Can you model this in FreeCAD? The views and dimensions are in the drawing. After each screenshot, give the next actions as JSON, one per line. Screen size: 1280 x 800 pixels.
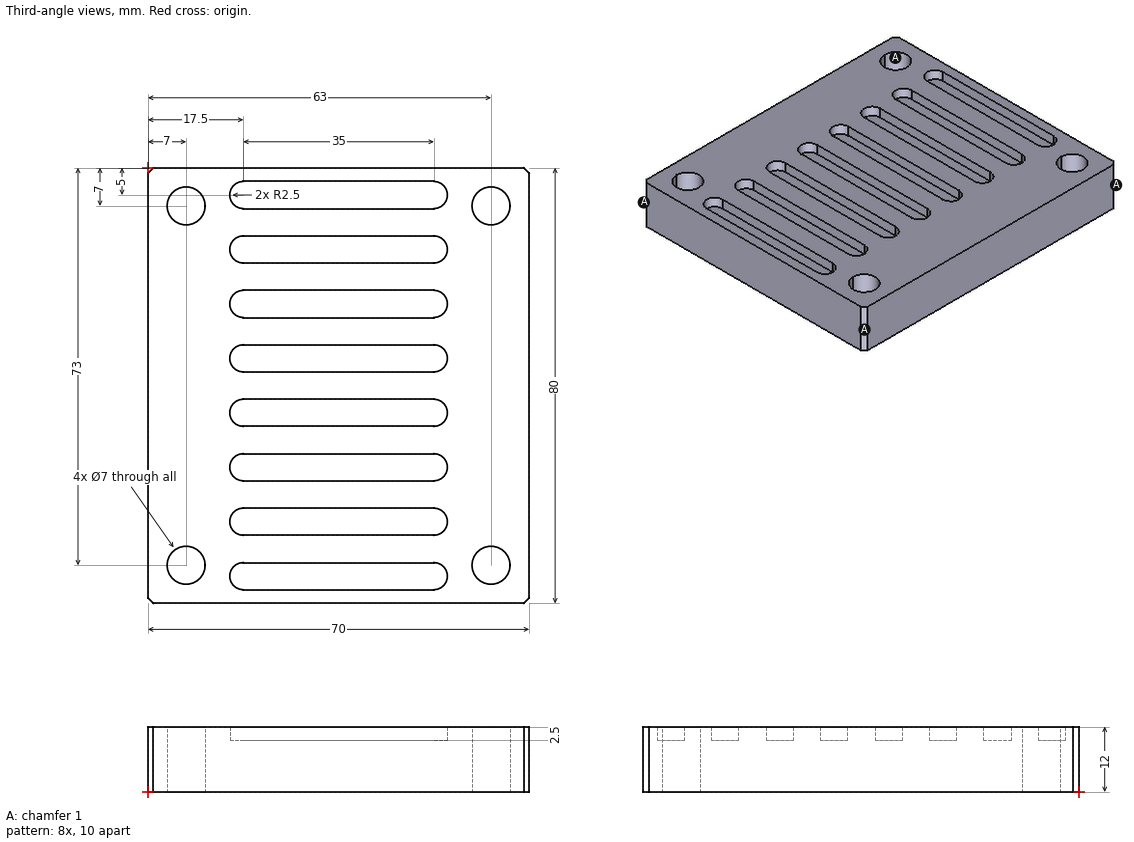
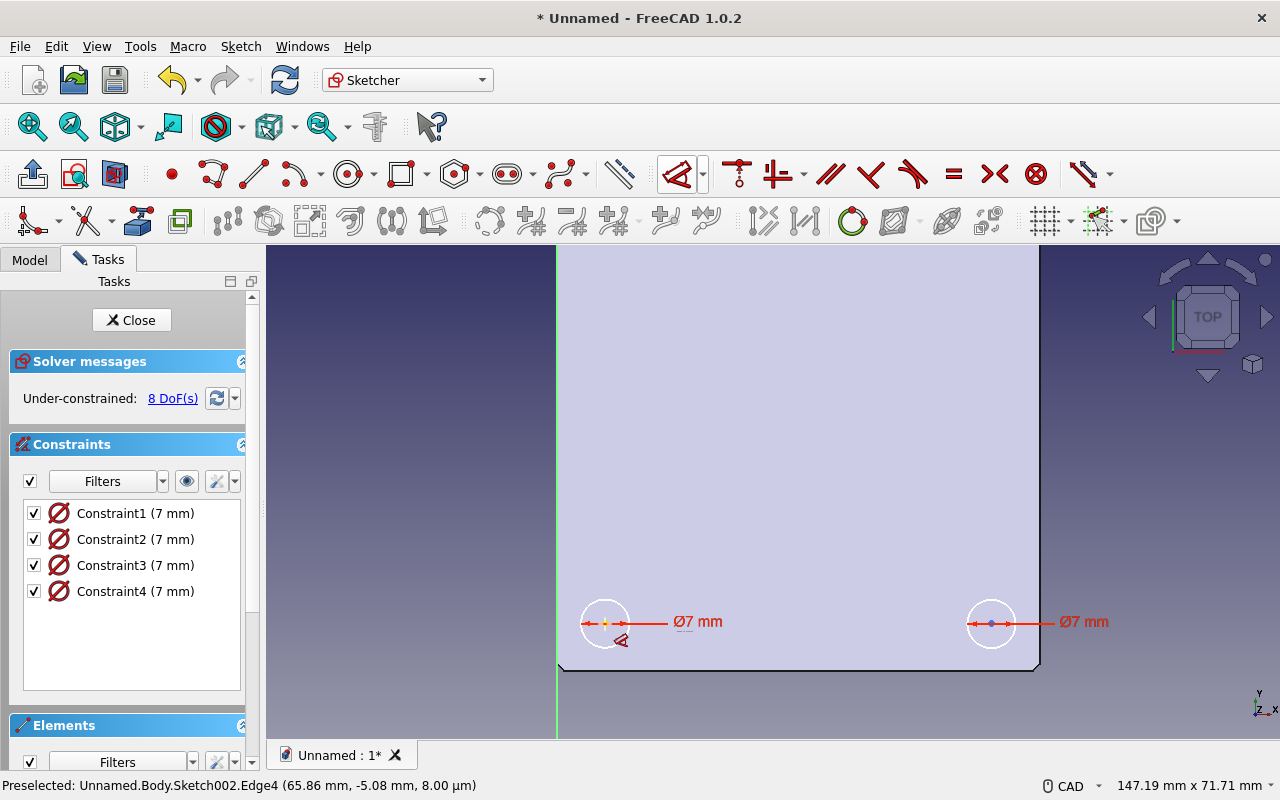
{"action": "left_click", "coordinate": [605, 624]}
{"action": "left_click", "coordinate": [581, 658]}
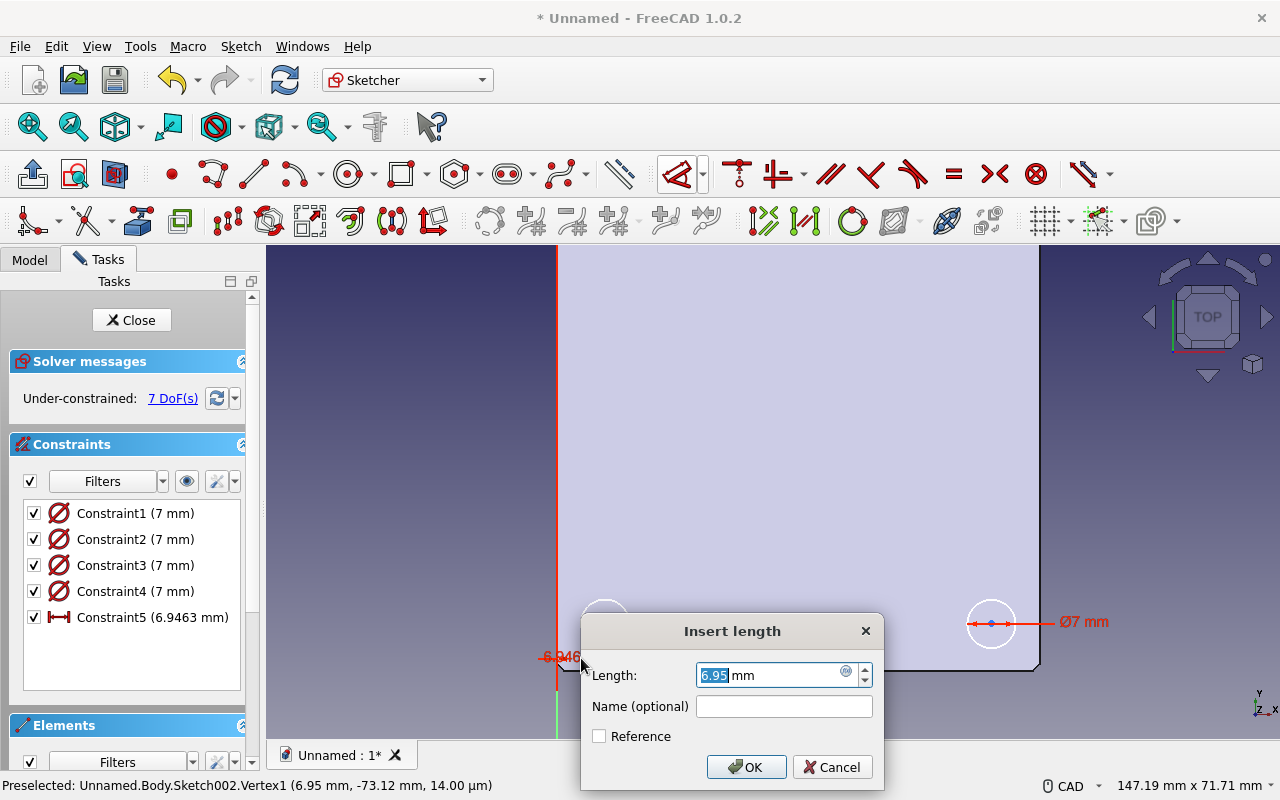
{"action": "type", "text": "7"}
{"action": "key", "text": "Return"}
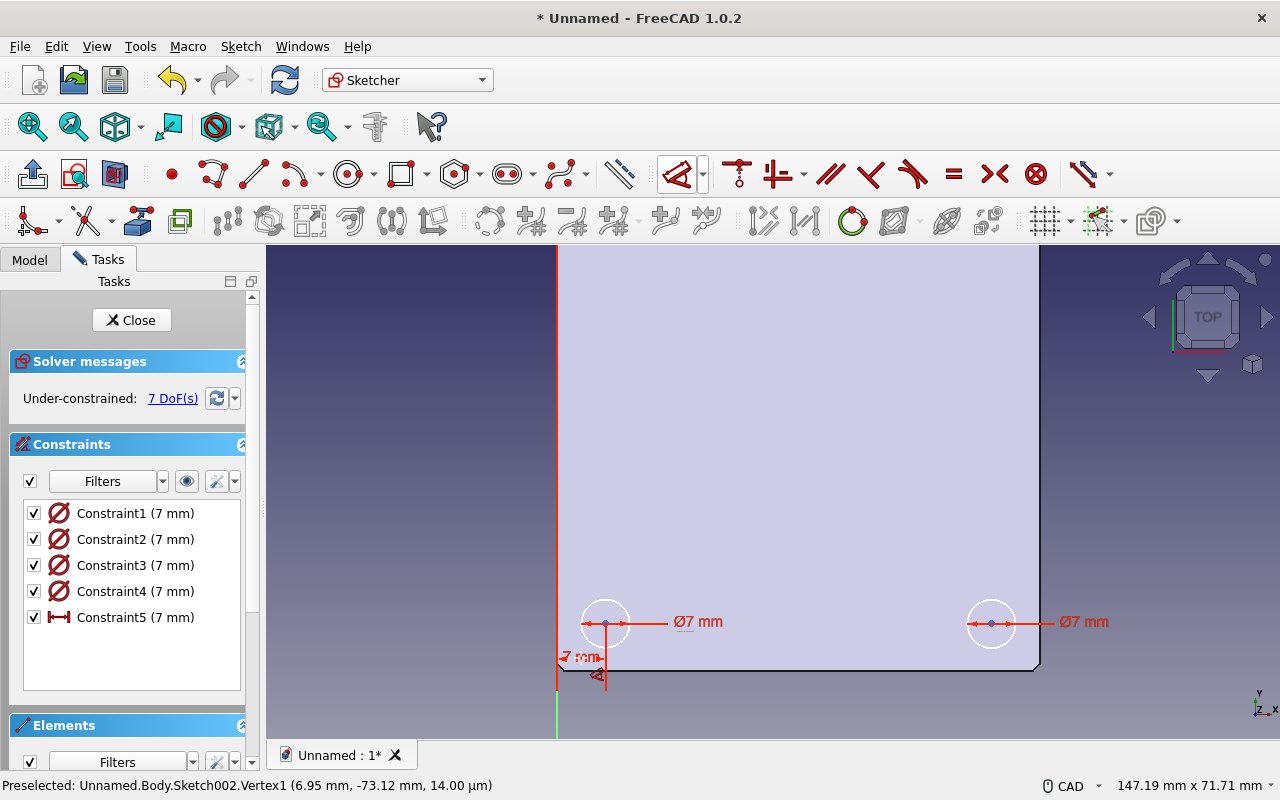
{"action": "scroll", "coordinate": [605, 624], "scroll_direction": "down", "scroll_amount": 3}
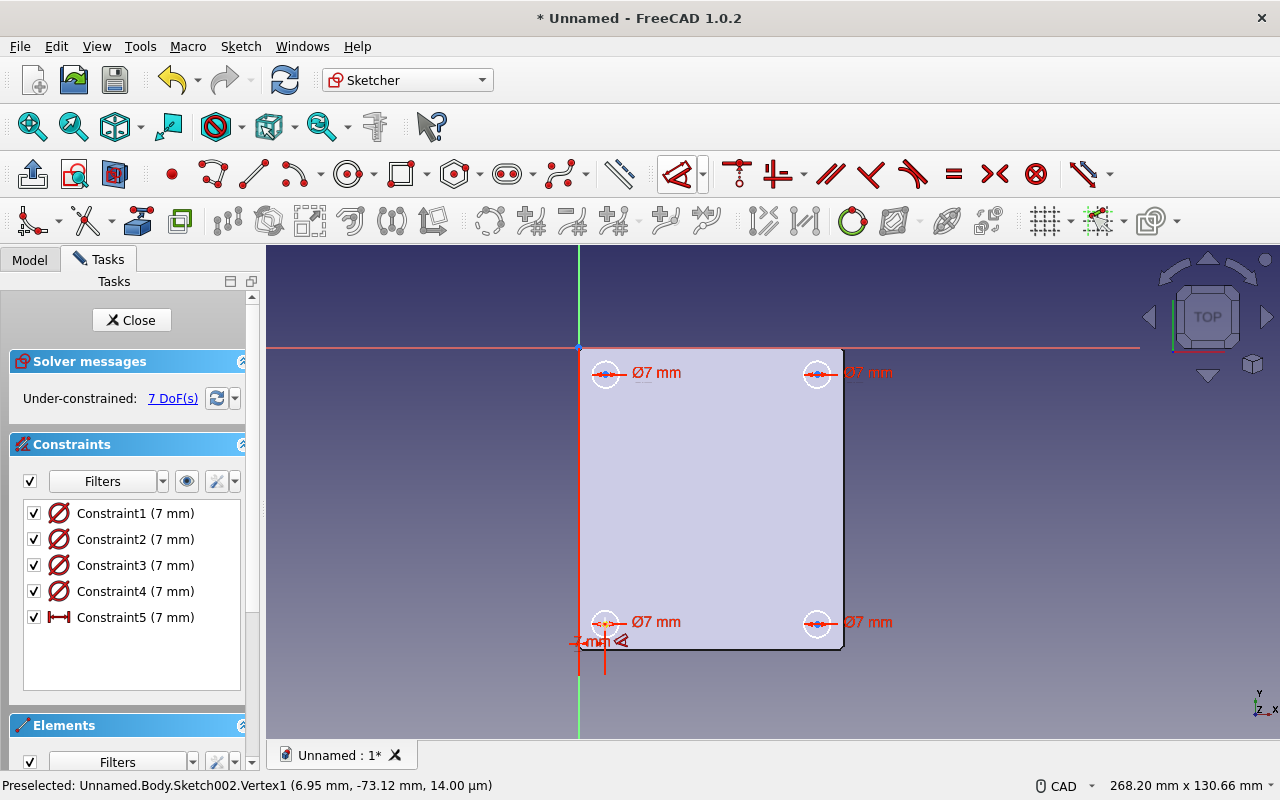
{"action": "scroll", "coordinate": [606, 375], "scroll_direction": "up", "scroll_amount": 3}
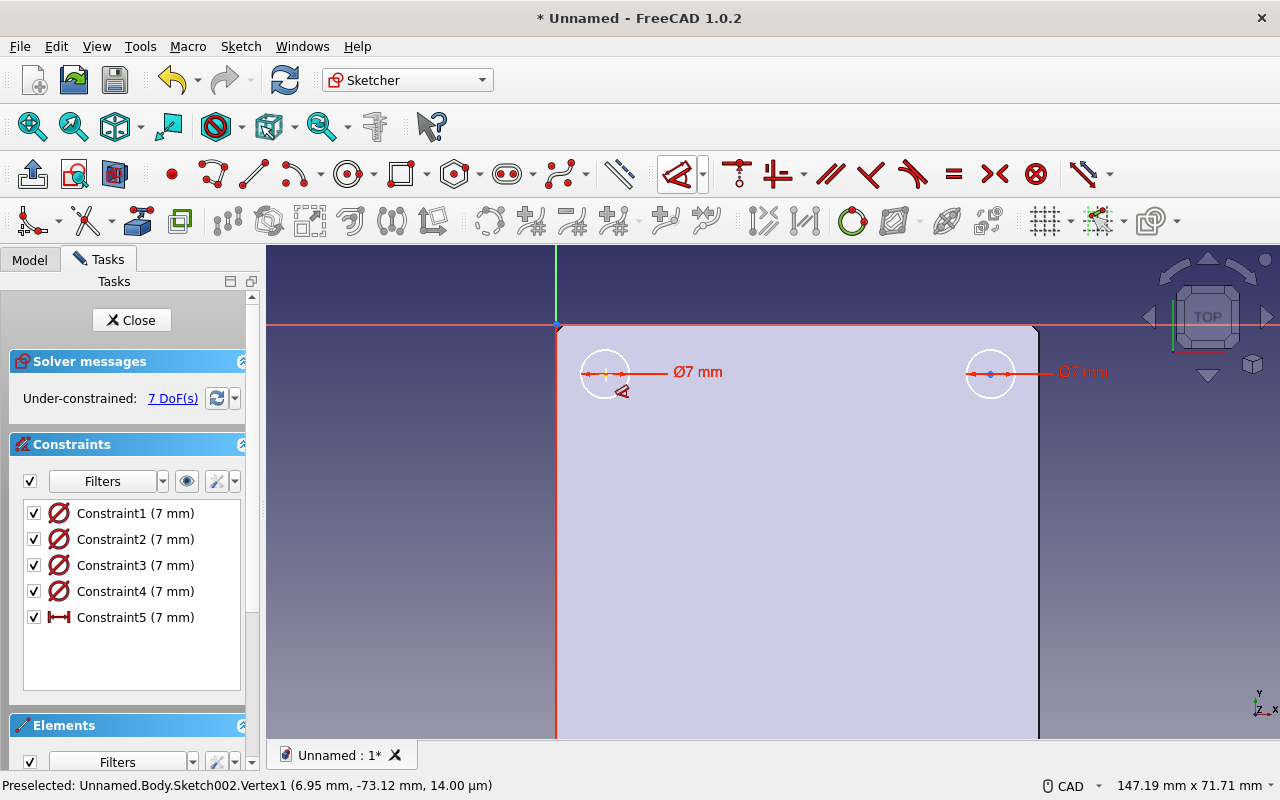
{"action": "left_click", "coordinate": [605, 374]}
{"action": "left_click", "coordinate": [581, 291]}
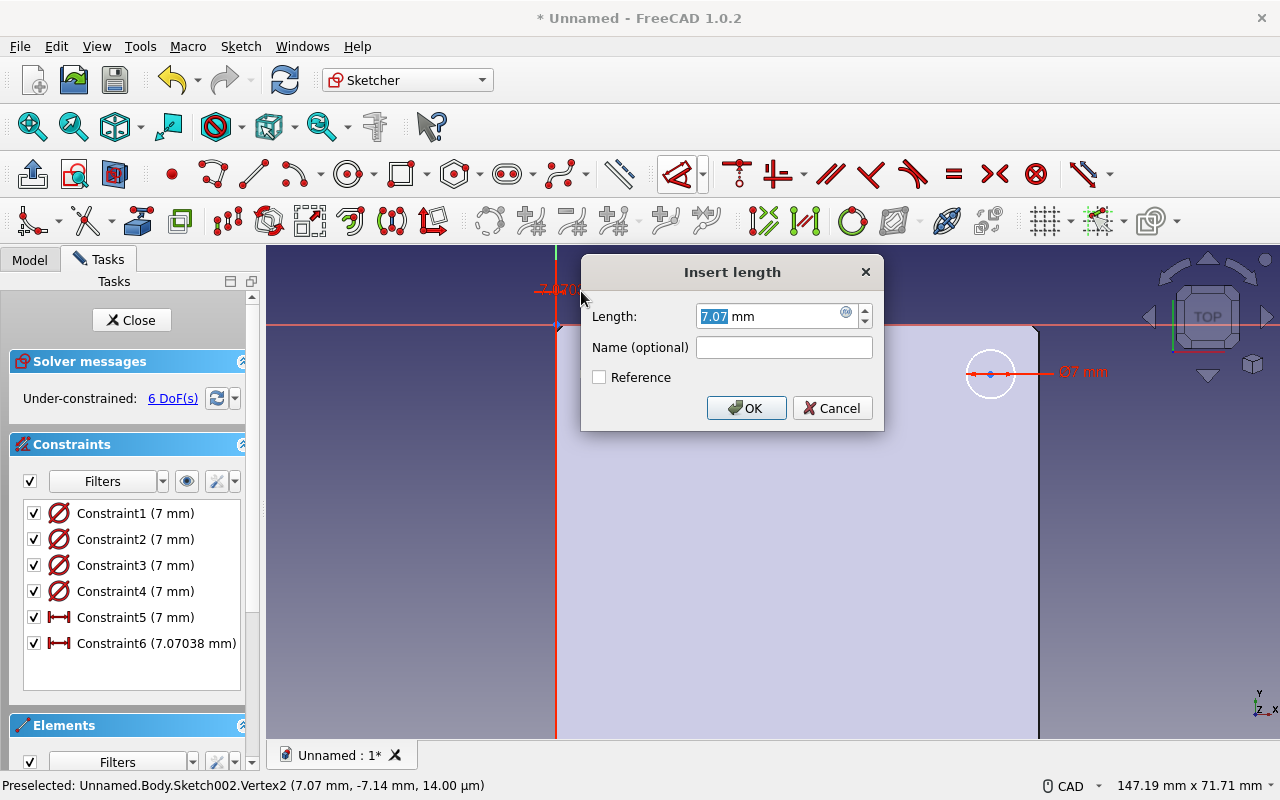
{"action": "type", "text": "7"}
{"action": "key", "text": "Return"}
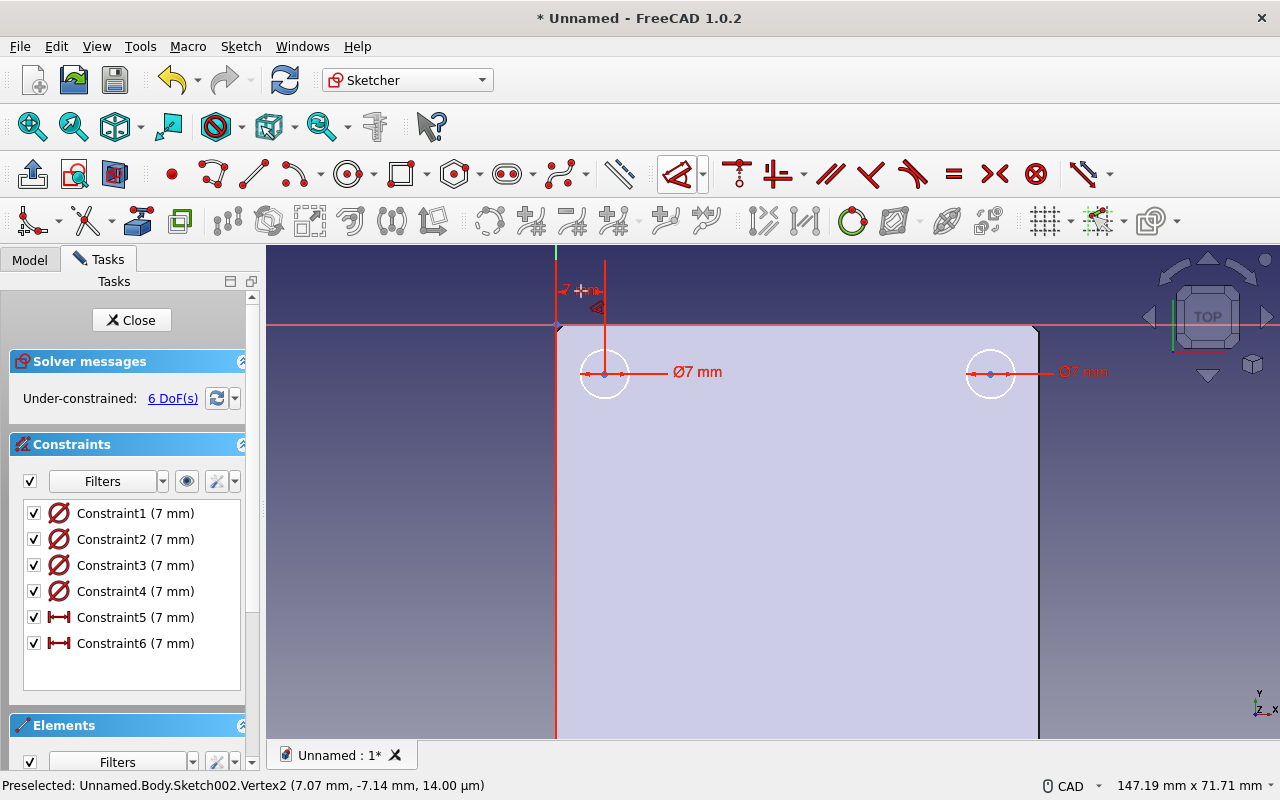
{"action": "left_click", "coordinate": [605, 374]}
{"action": "left_click", "coordinate": [522, 350]}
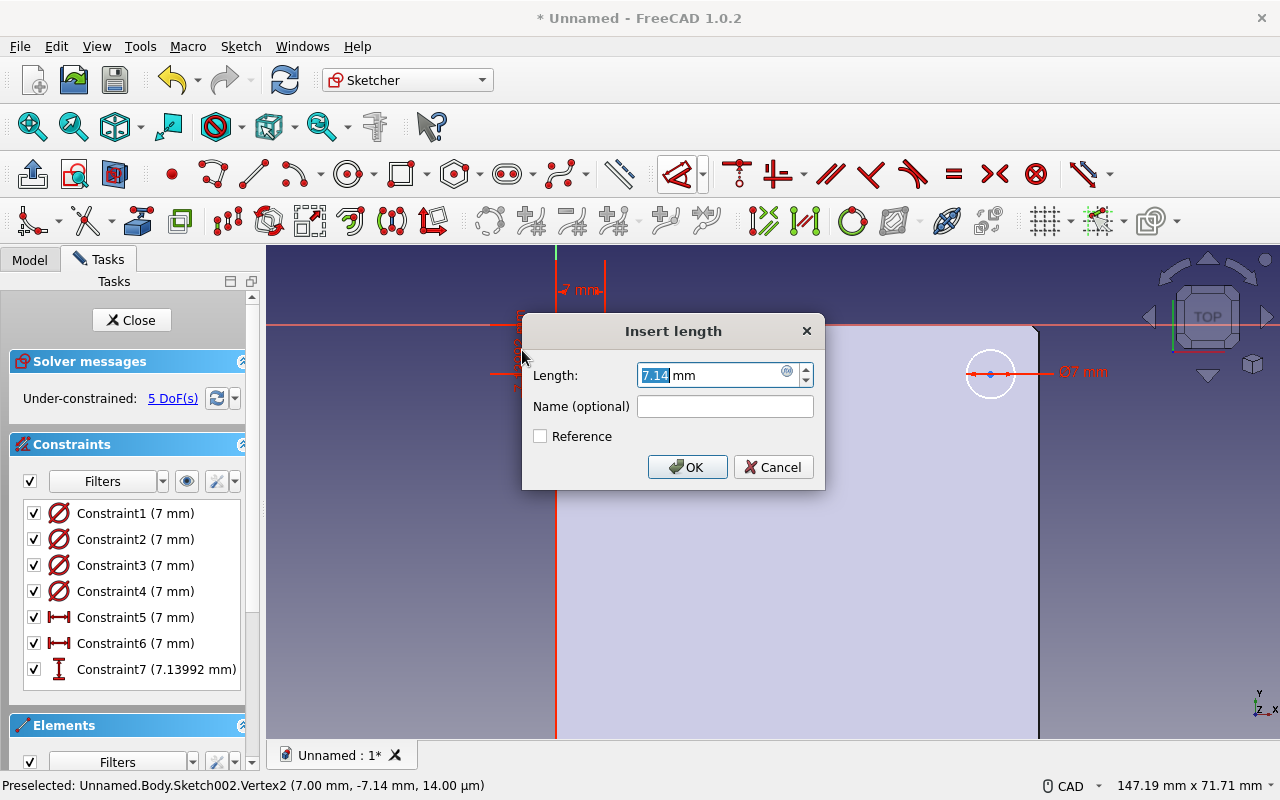
{"action": "type", "text": "7"}
{"action": "key", "text": "Return"}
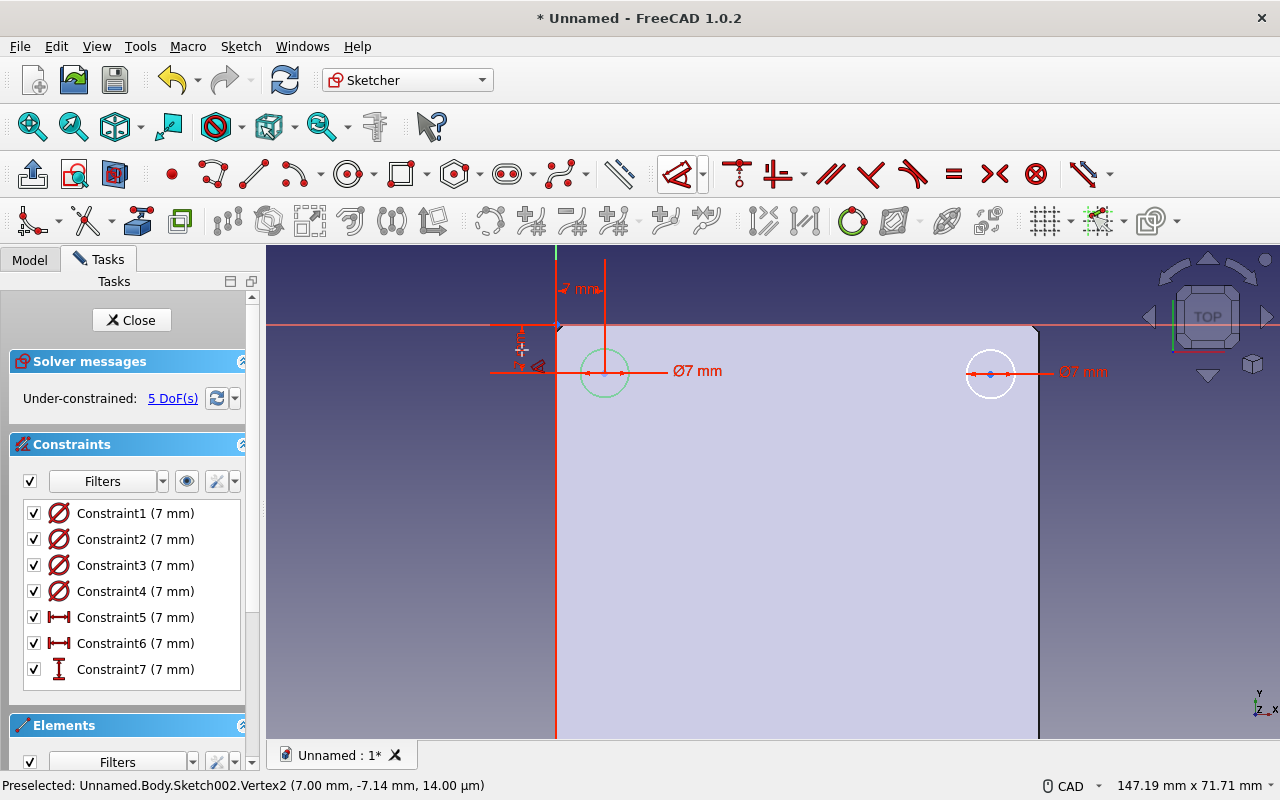
{"action": "left_click", "coordinate": [991, 374]}
{"action": "left_click", "coordinate": [1025, 350]}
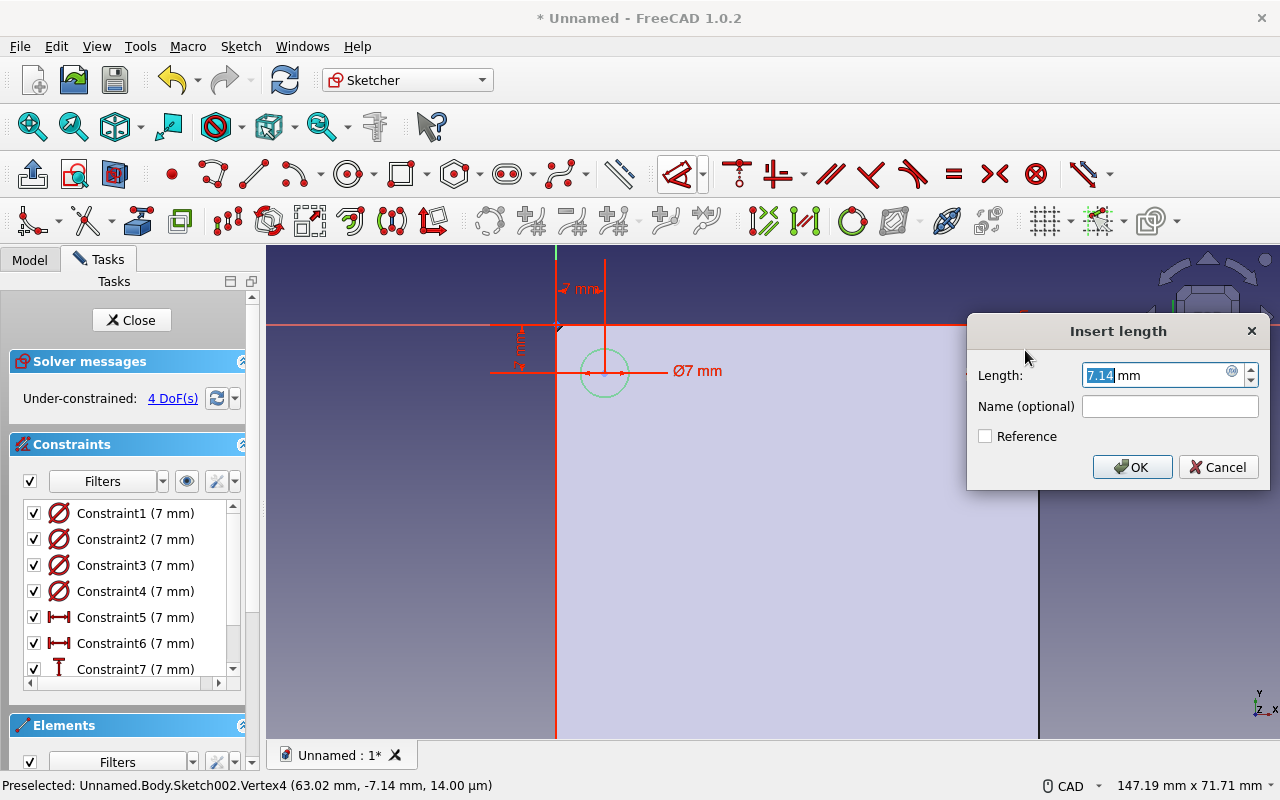
{"action": "type", "text": "7"}
{"action": "key", "text": "Return"}